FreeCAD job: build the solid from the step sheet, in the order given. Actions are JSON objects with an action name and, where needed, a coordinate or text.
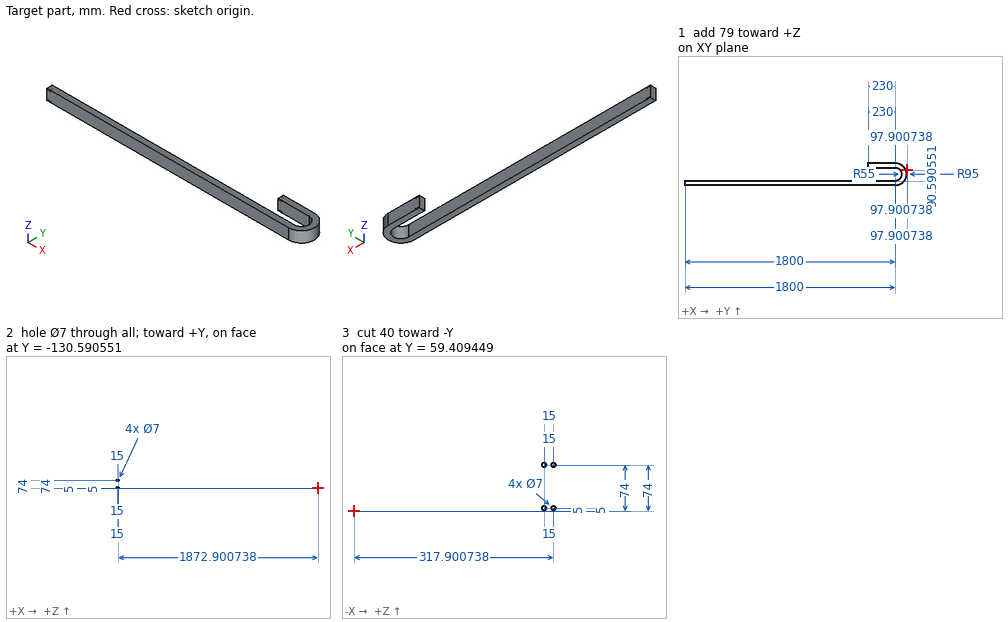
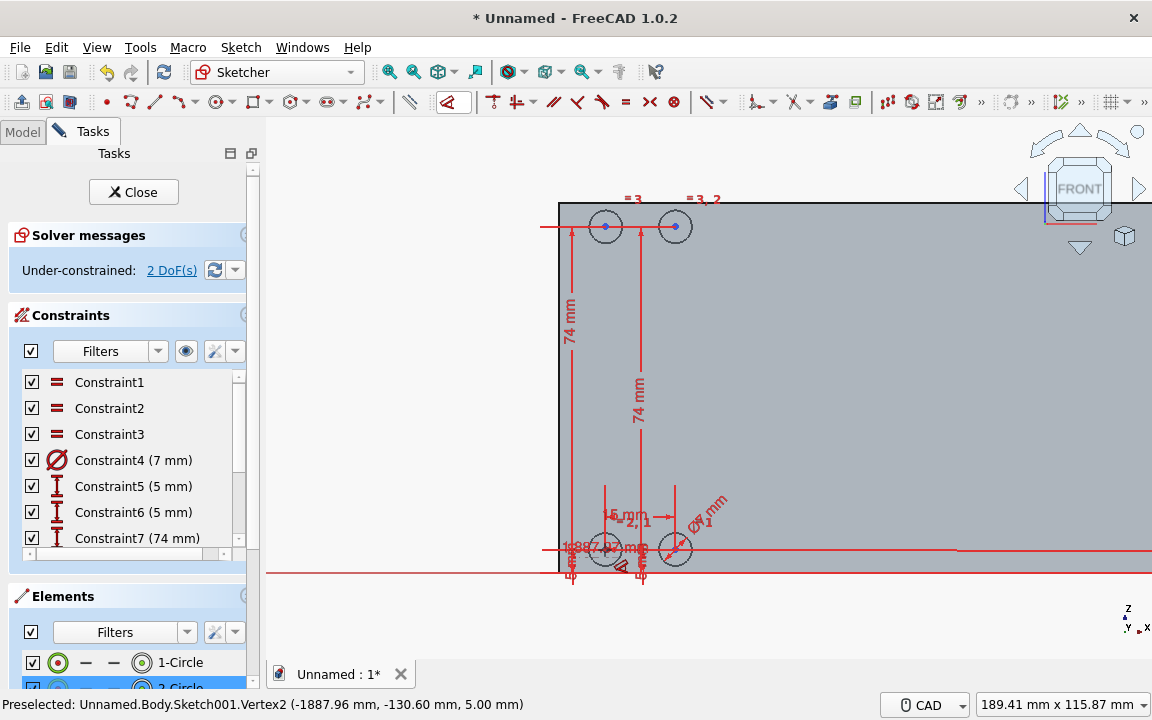
{"action": "left_click", "coordinate": [675, 227]}
{"action": "left_click", "coordinate": [640, 193]}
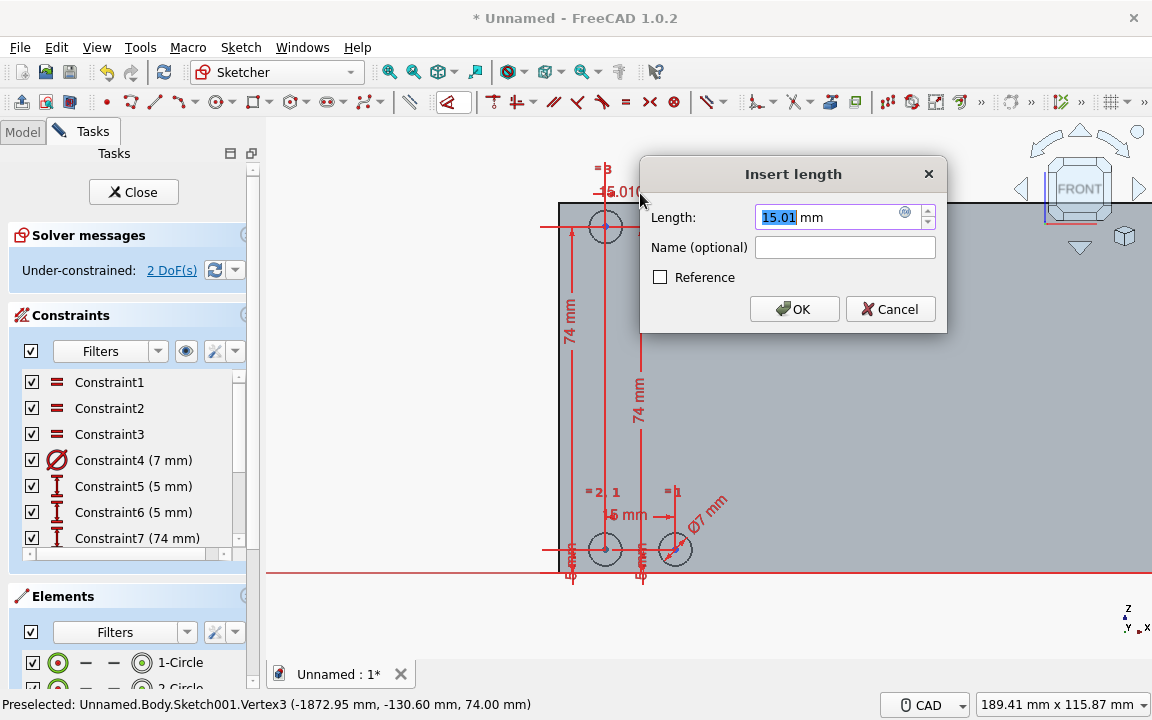
{"action": "type", "text": "15"}
{"action": "key", "text": "Return"}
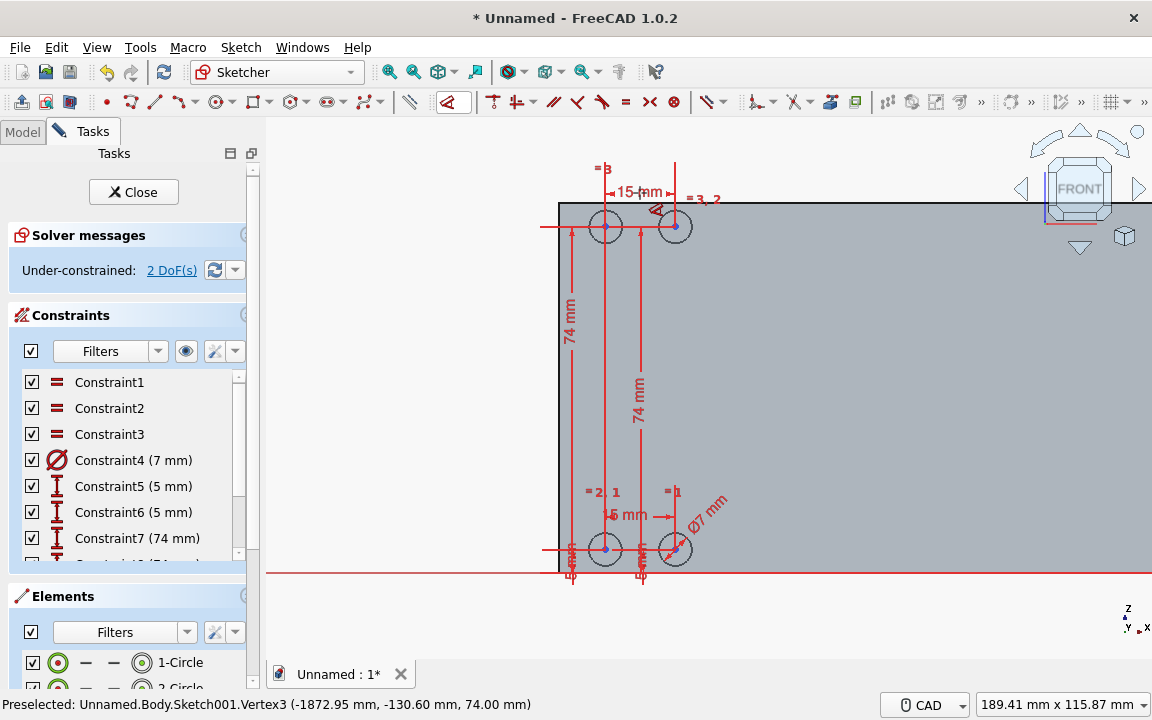
{"action": "left_click", "coordinate": [675, 227]}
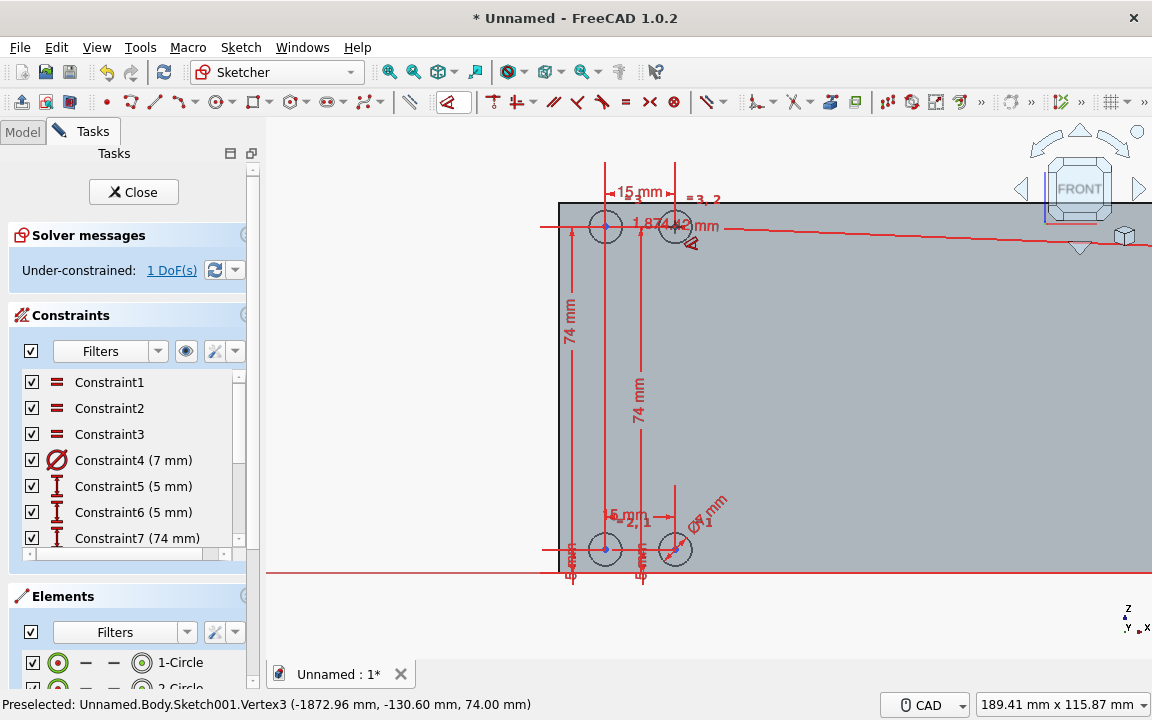
{"action": "left_click", "coordinate": [606, 227]}
{"action": "left_click", "coordinate": [641, 261]}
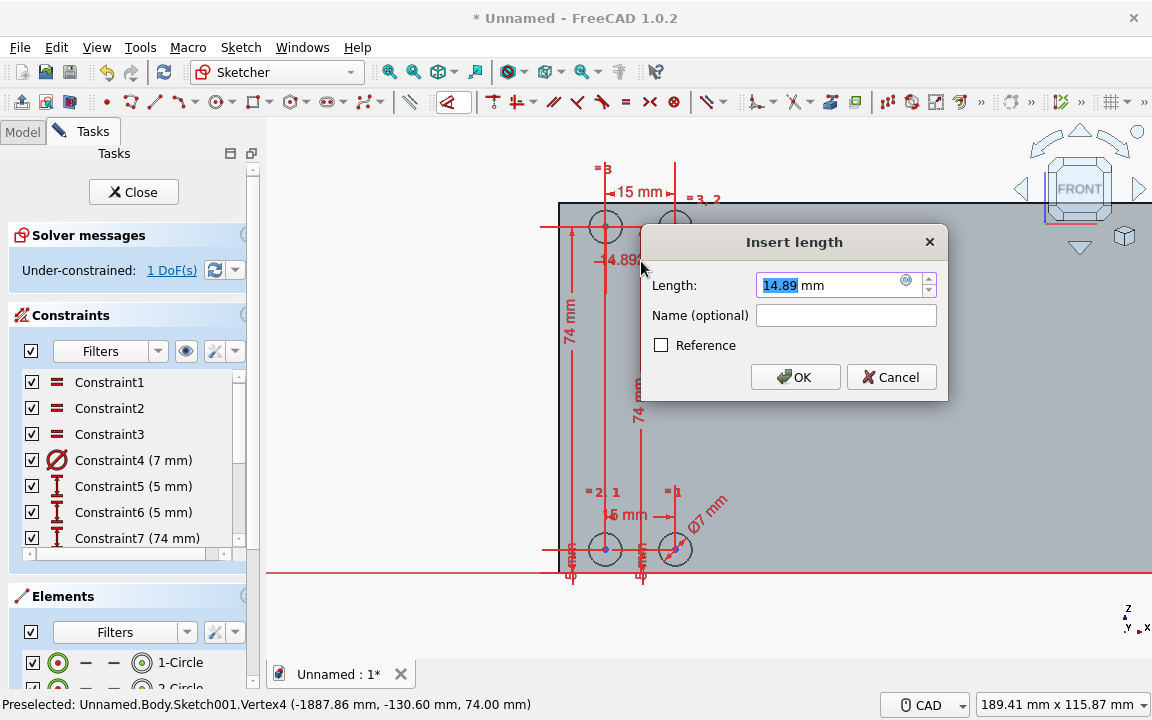
{"action": "type", "text": "15"}
{"action": "key", "text": "Return"}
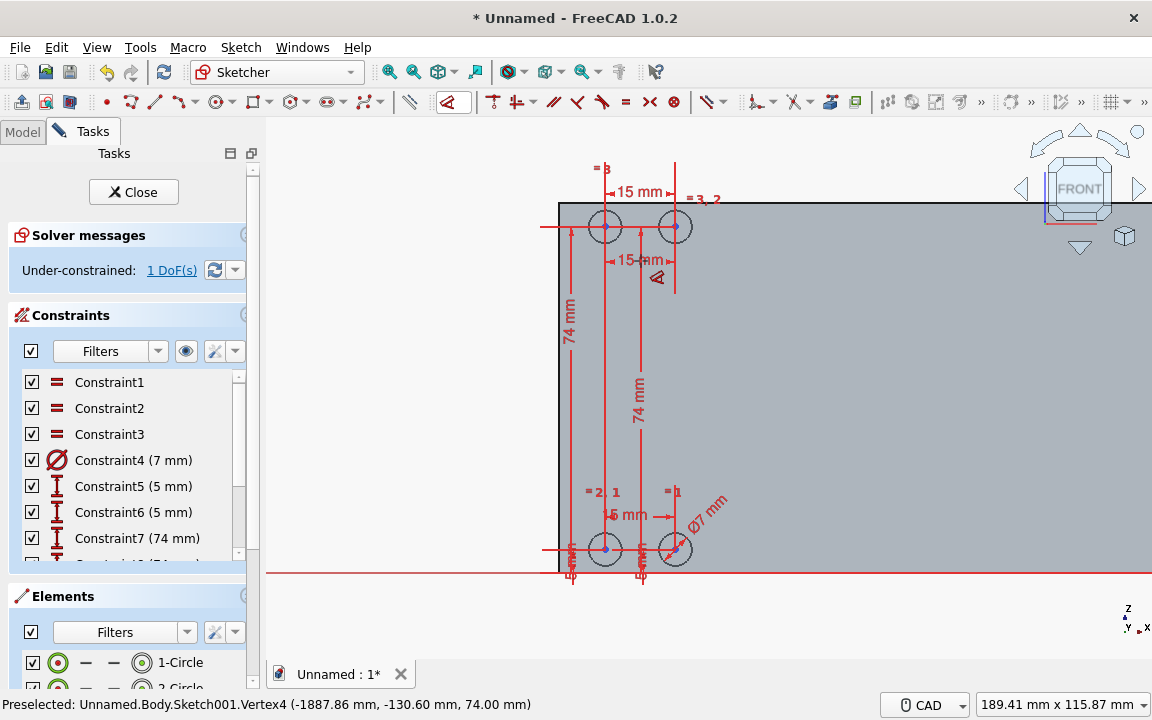
{"action": "left_click", "coordinate": [675, 550]}
{"action": "left_click", "coordinate": [831, 607]}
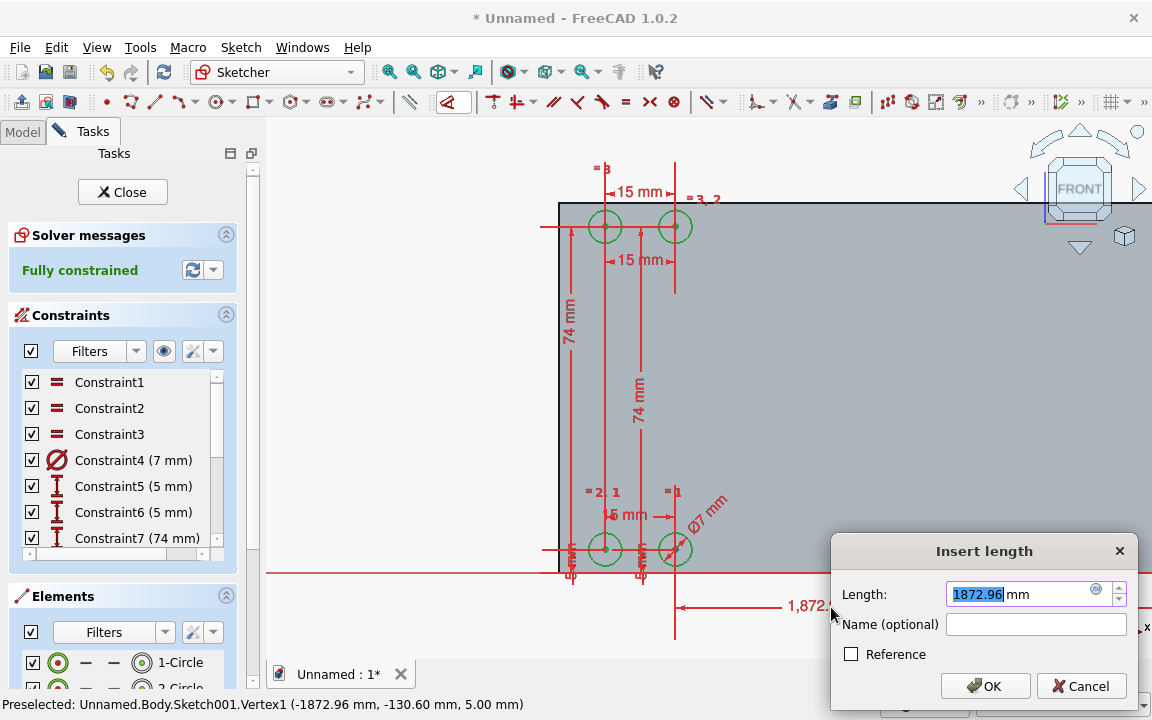
{"action": "type", "text": "1872.900738"}
{"action": "key", "text": "Return"}
{"action": "key", "text": "Escape"}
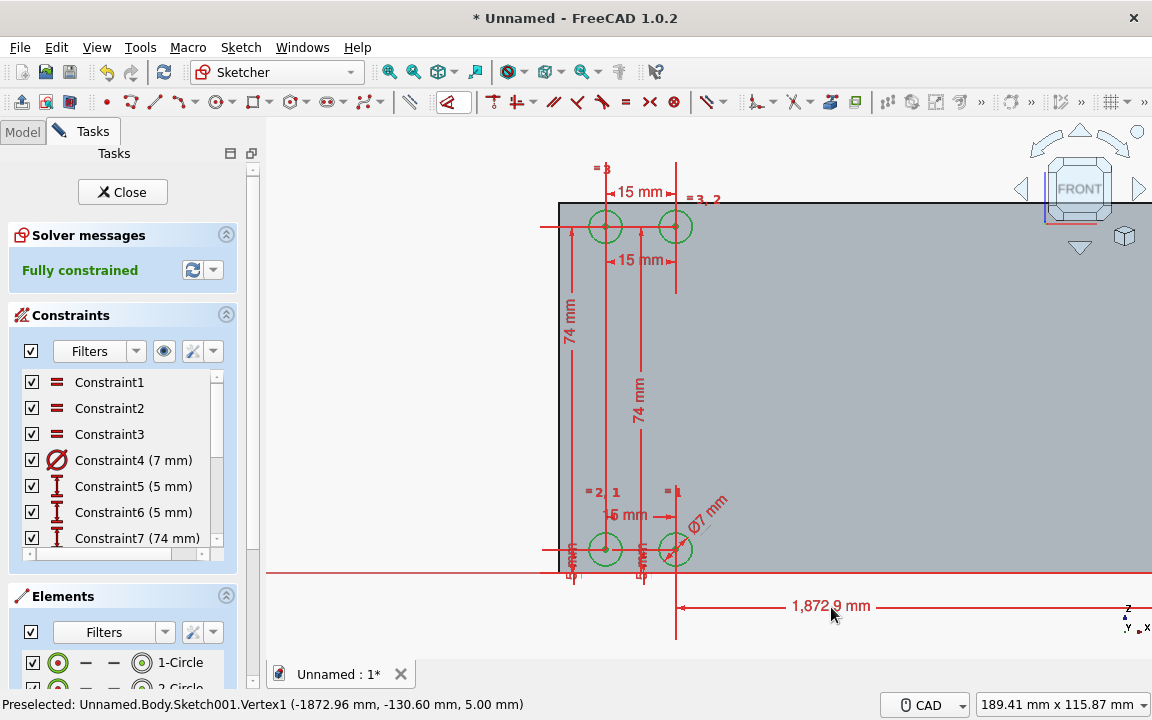
{"action": "left_click", "coordinate": [123, 192]}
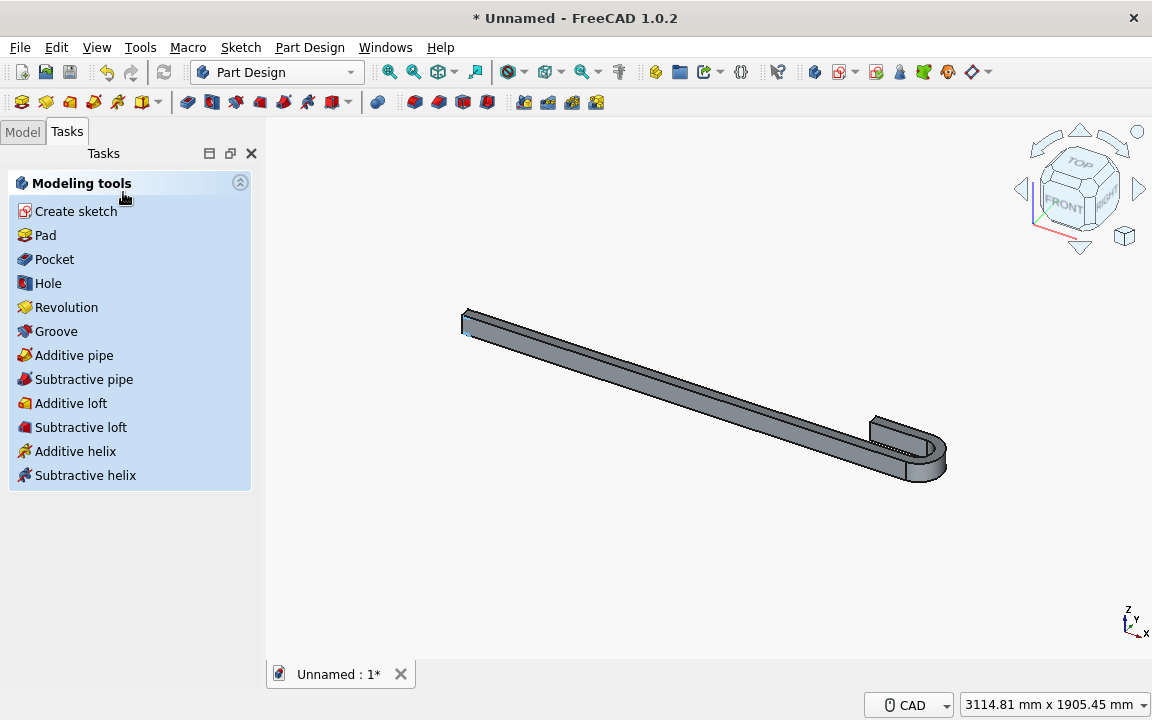
{"action": "left_click", "coordinate": [212, 102]}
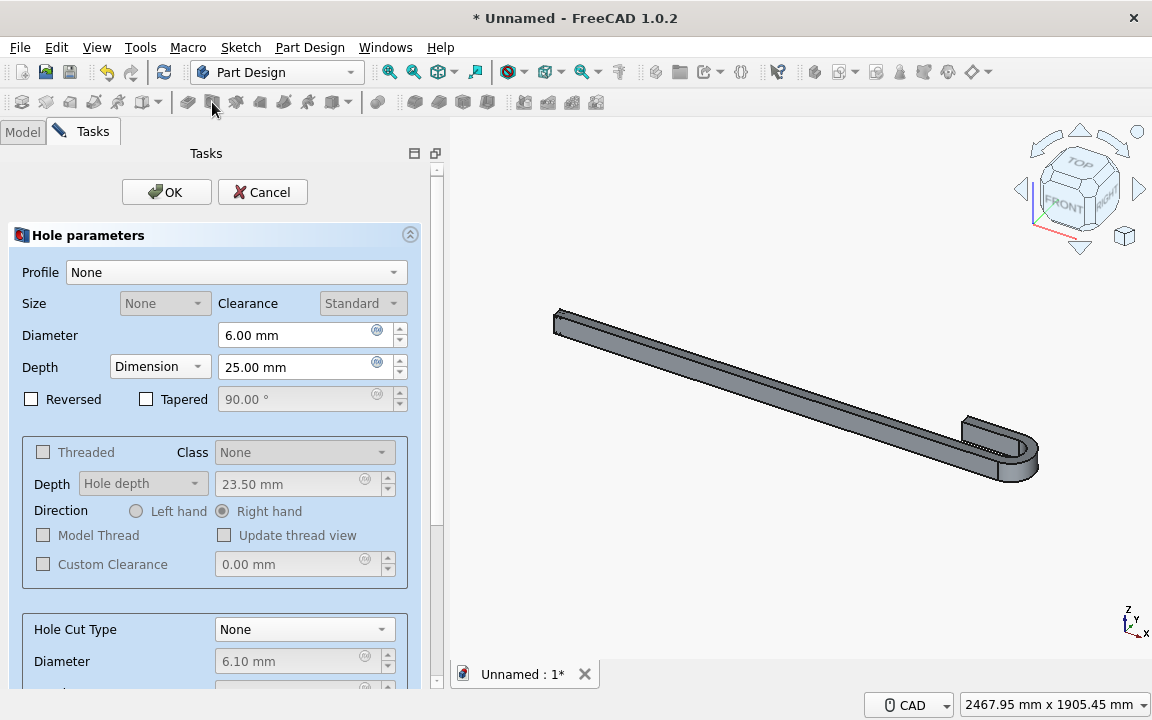
{"action": "triple_click", "coordinate": [305, 335]}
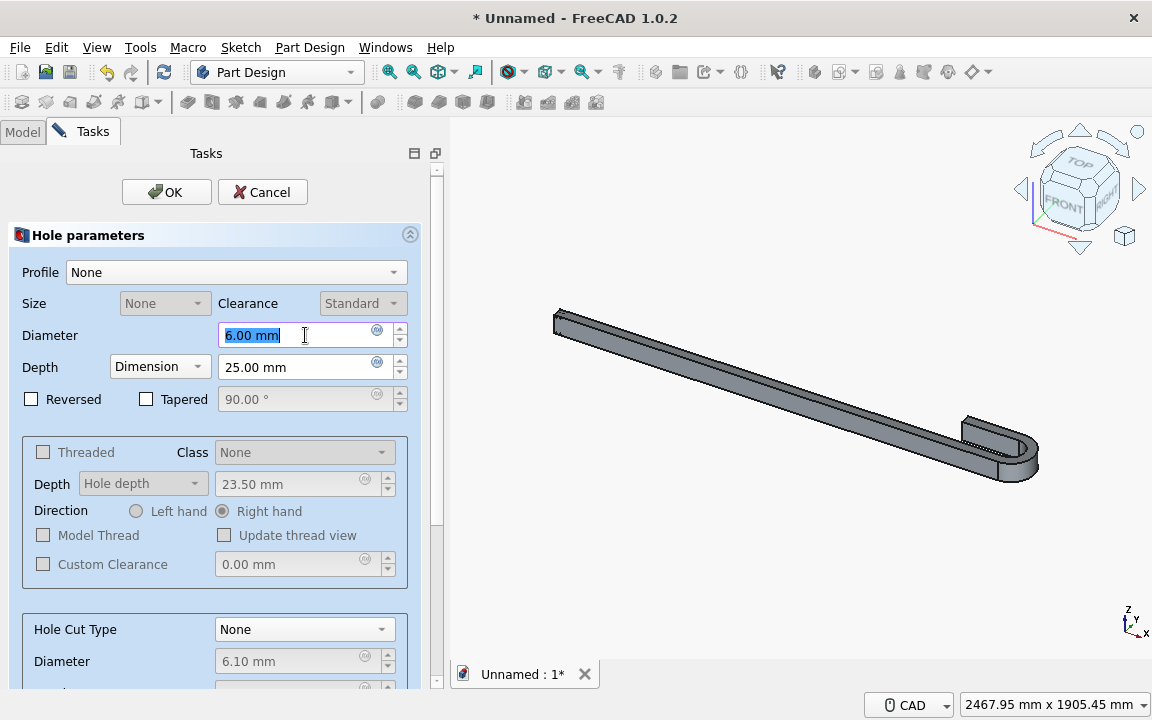
{"action": "type", "text": "7"}
{"action": "key", "text": "Tab"}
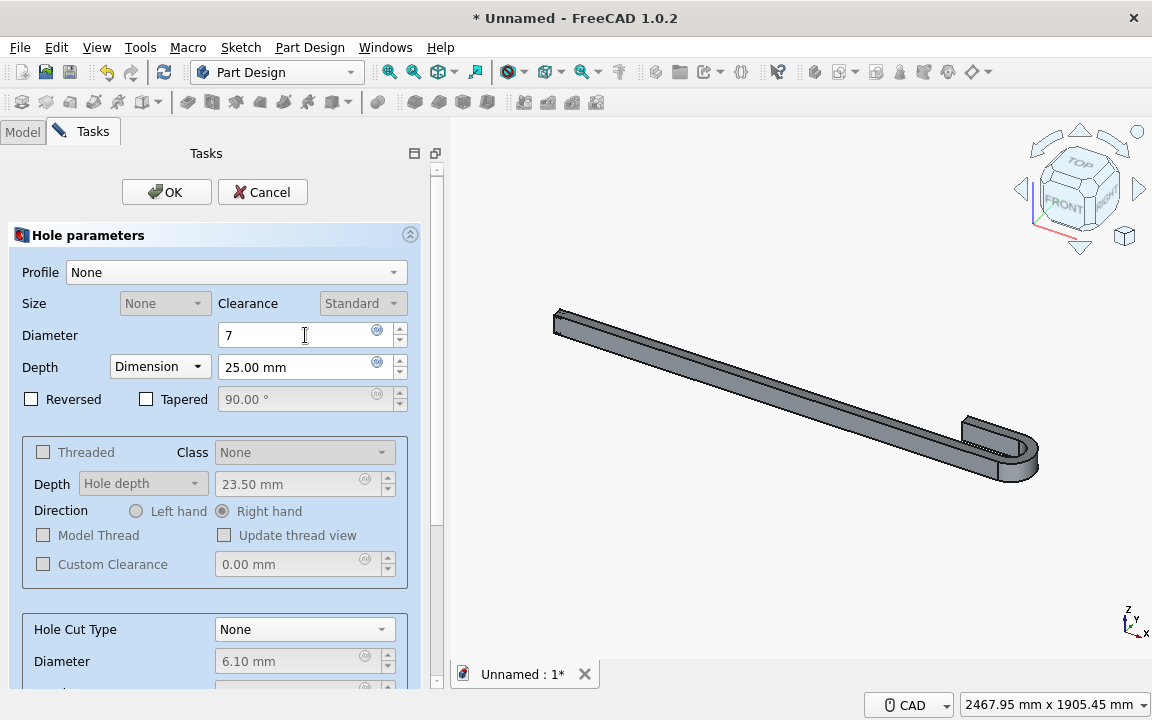
{"action": "left_click", "coordinate": [161, 366]}